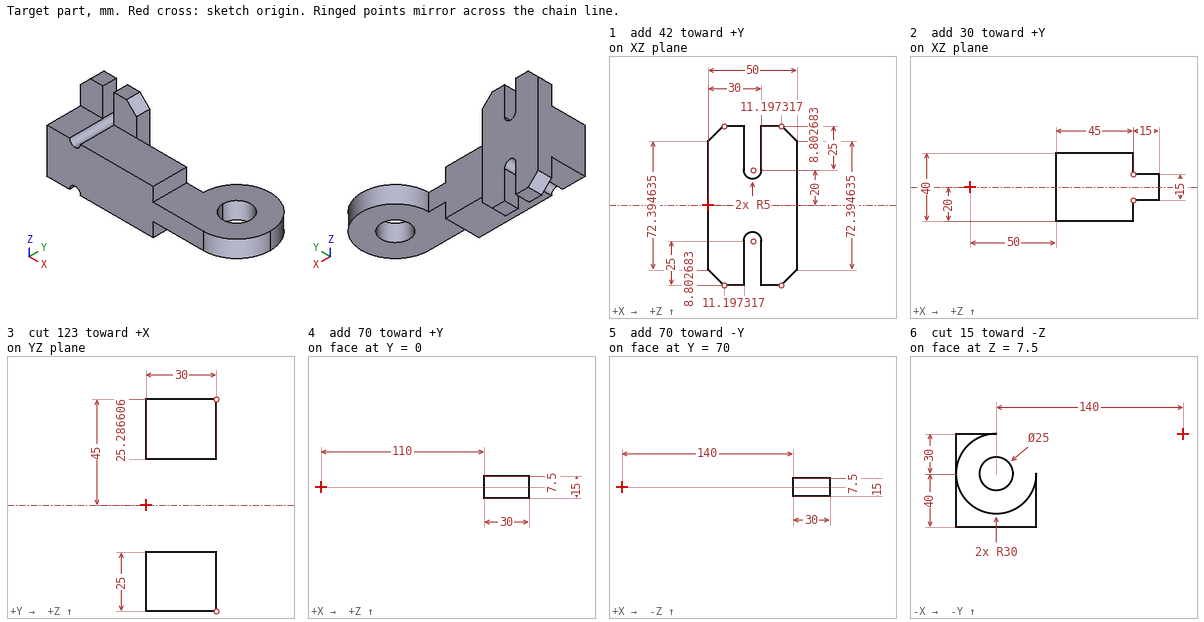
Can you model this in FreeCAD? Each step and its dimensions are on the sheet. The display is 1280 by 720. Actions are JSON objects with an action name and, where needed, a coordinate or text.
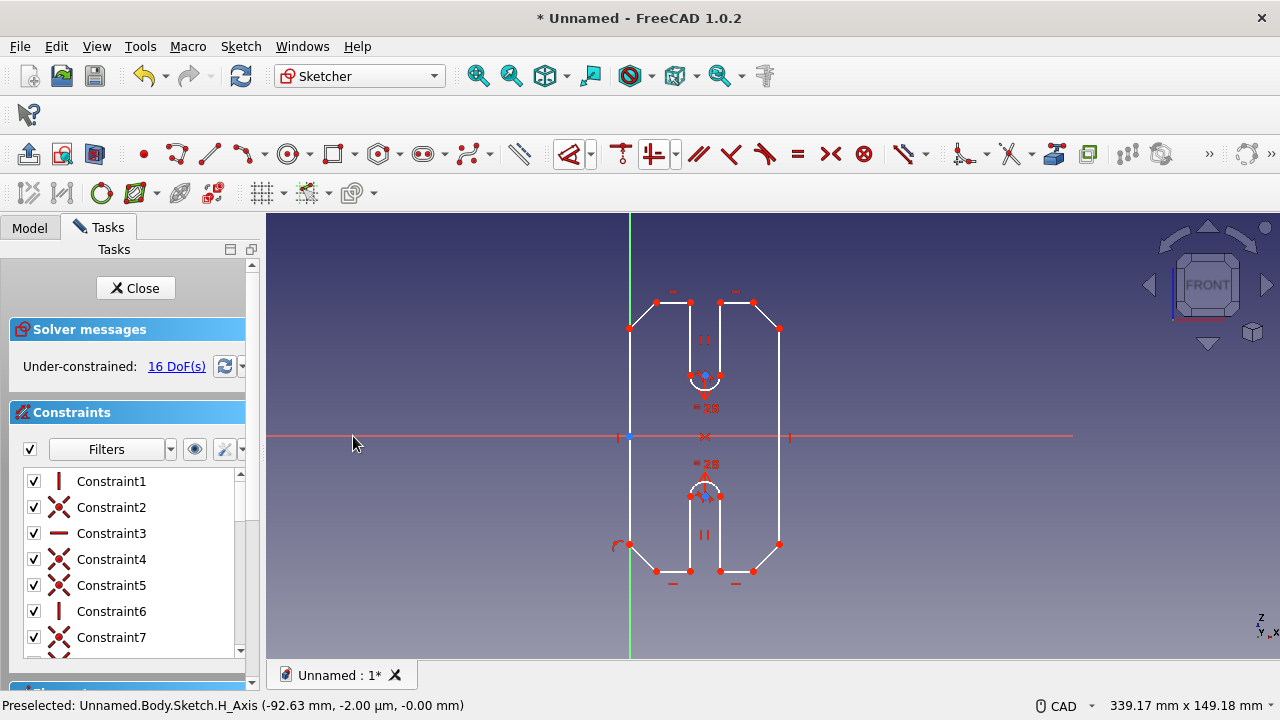
{"action": "left_click", "coordinate": [753, 303]}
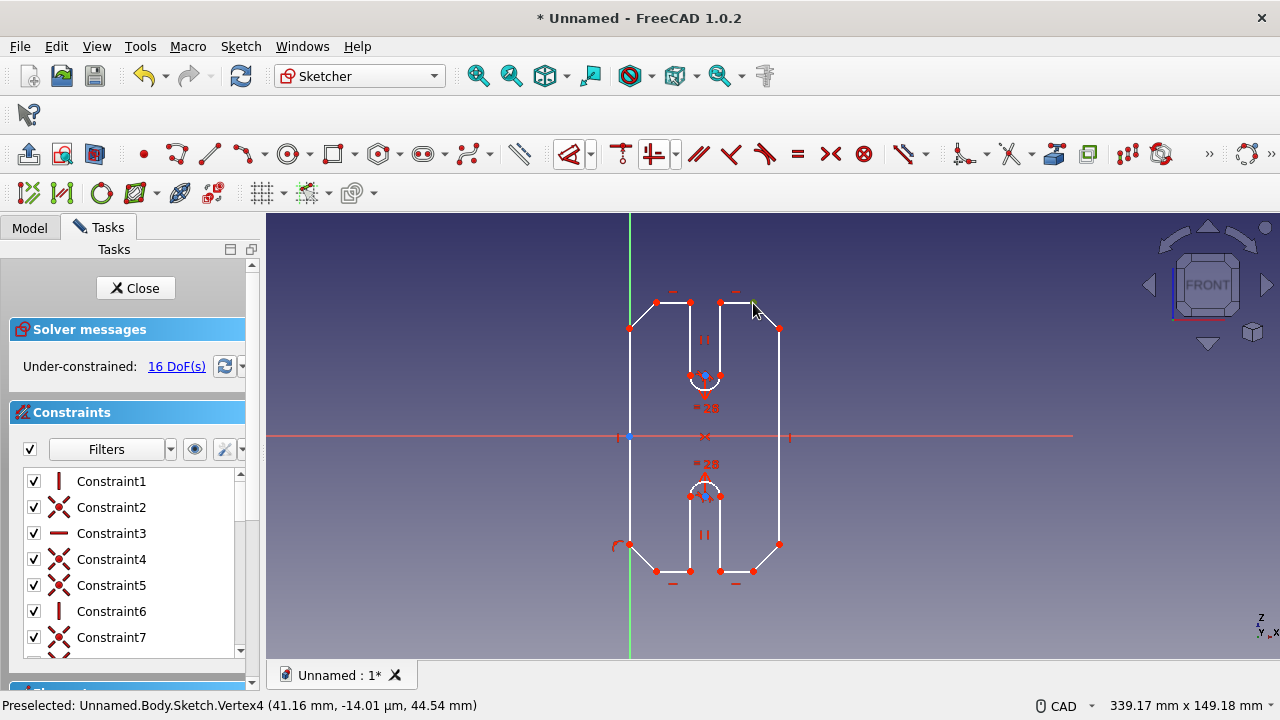
{"action": "left_click", "coordinate": [753, 572]}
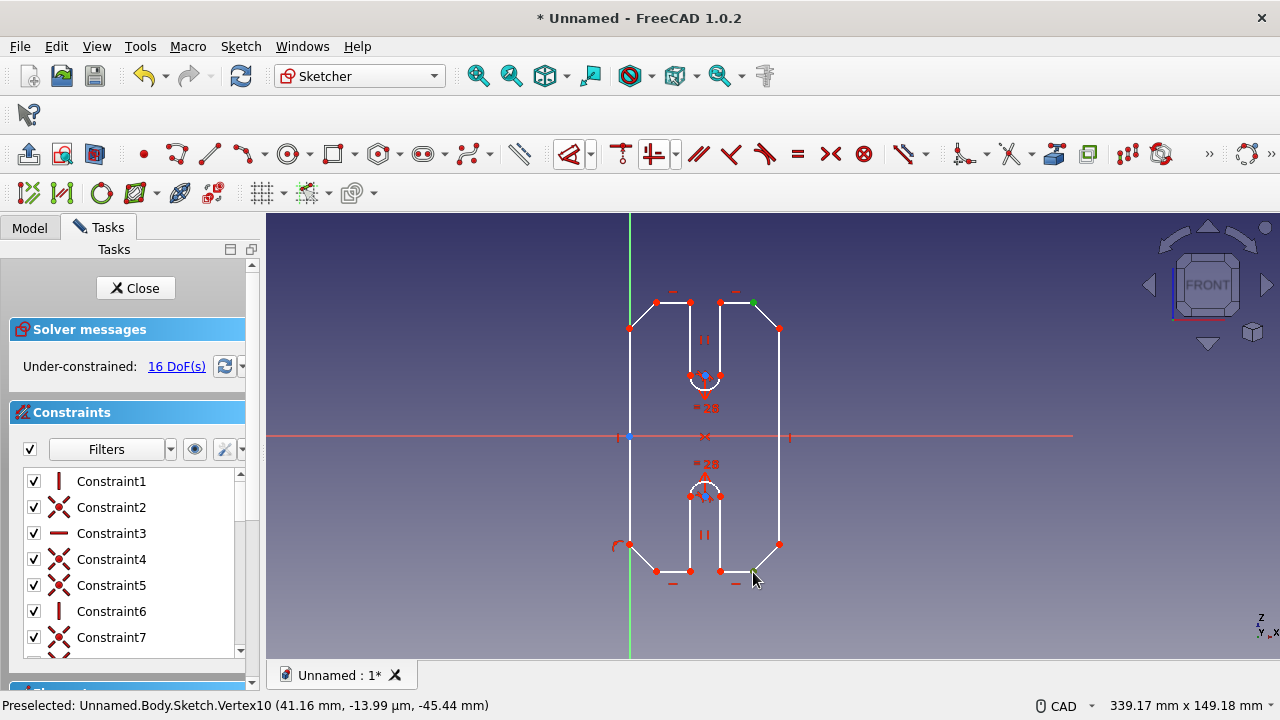
{"action": "left_click", "coordinate": [353, 436]}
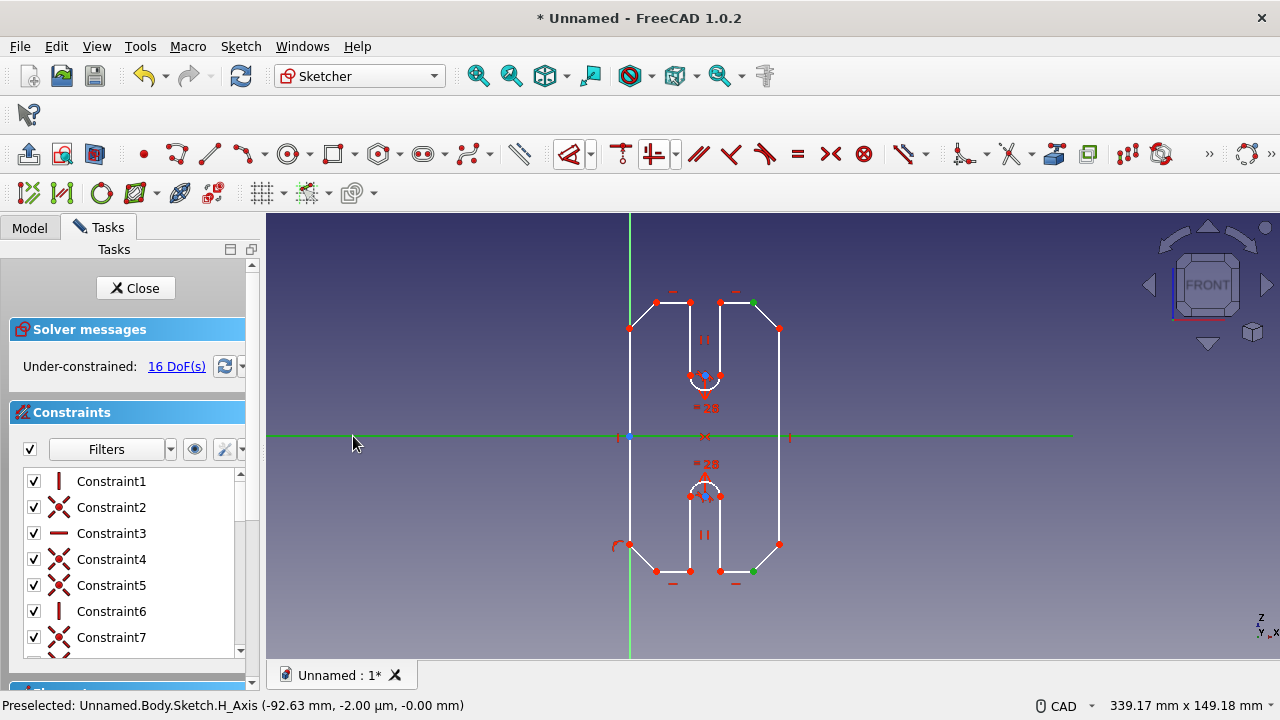
{"action": "left_click", "coordinate": [831, 154]}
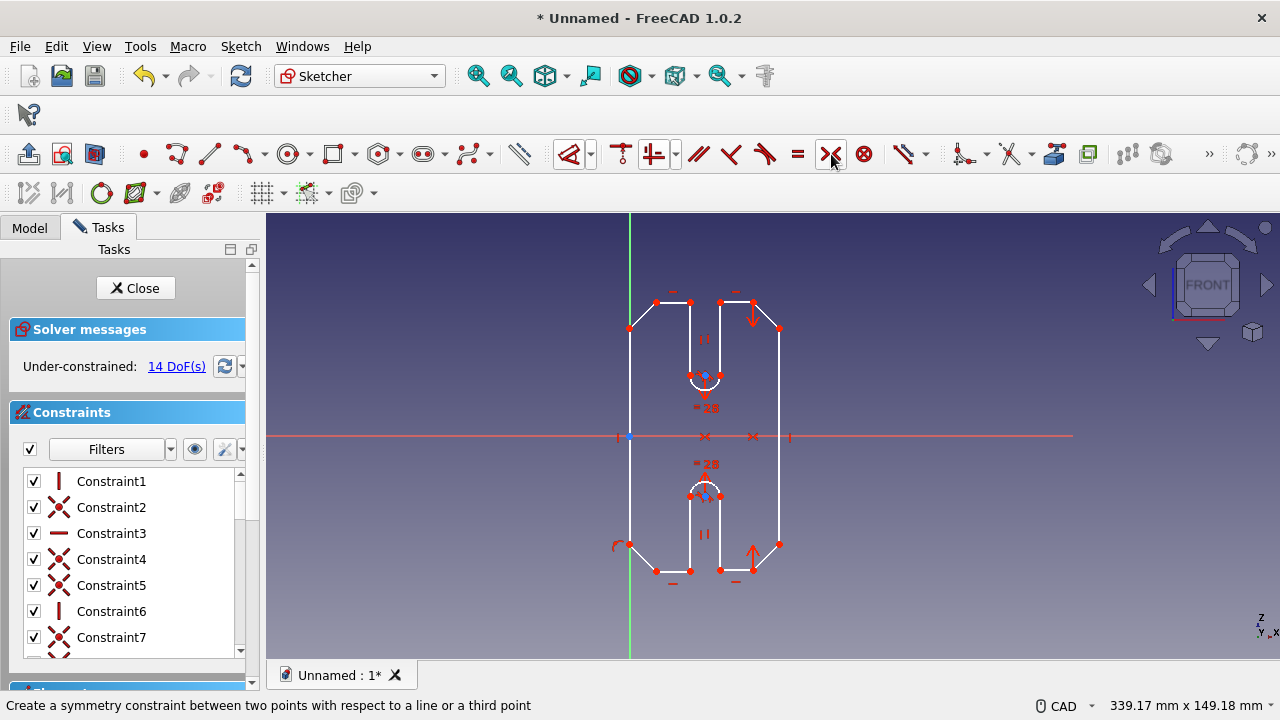
{"action": "left_click", "coordinate": [656, 572]}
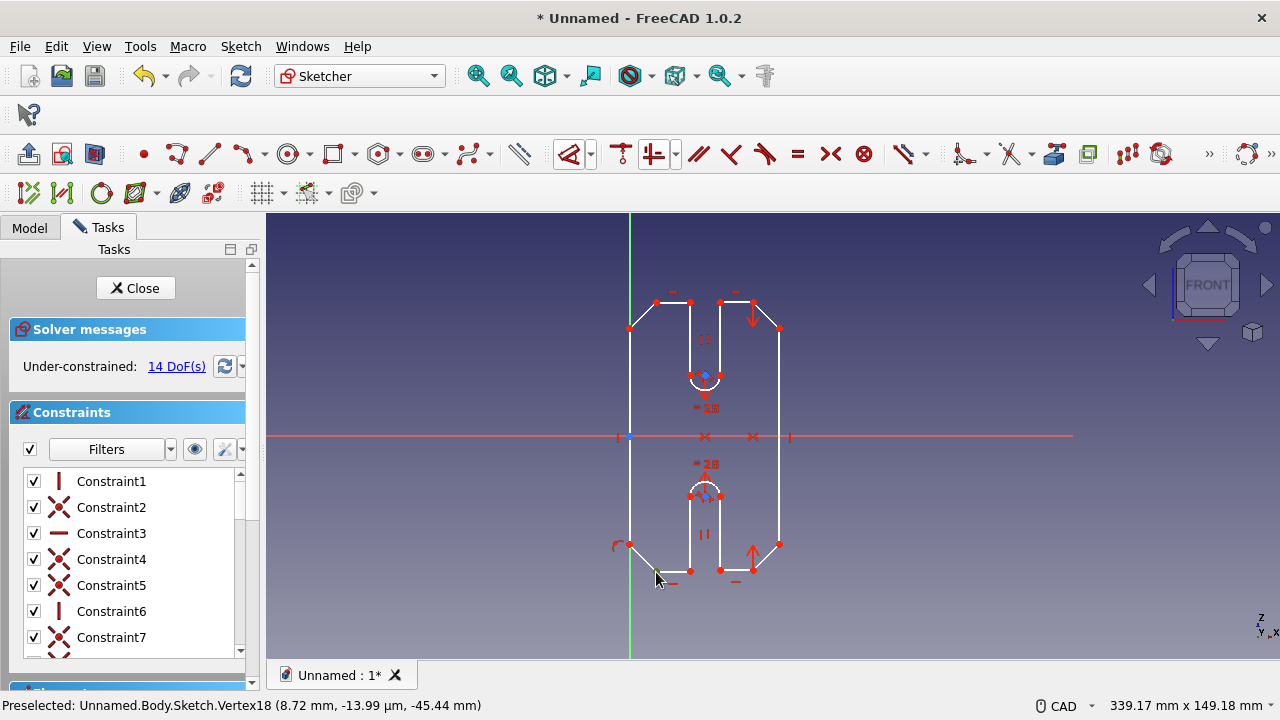
{"action": "left_click", "coordinate": [656, 303]}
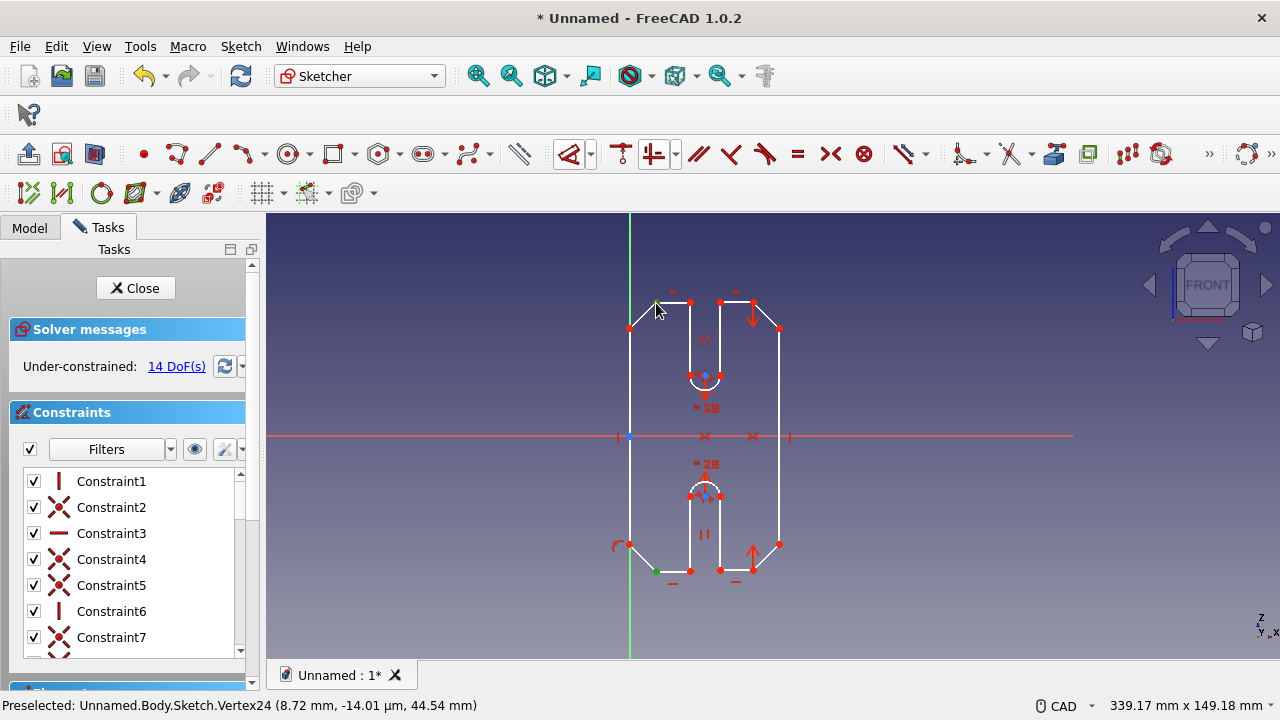
{"action": "left_click", "coordinate": [353, 436]}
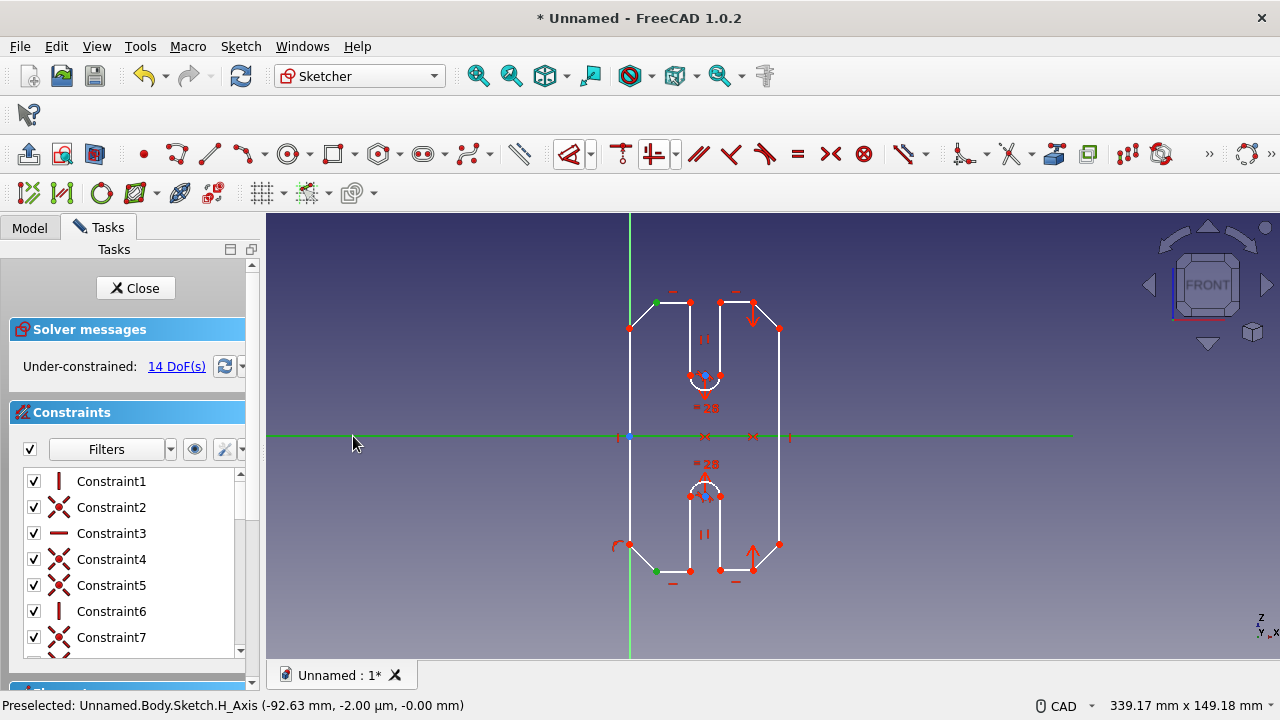
{"action": "left_click", "coordinate": [831, 154]}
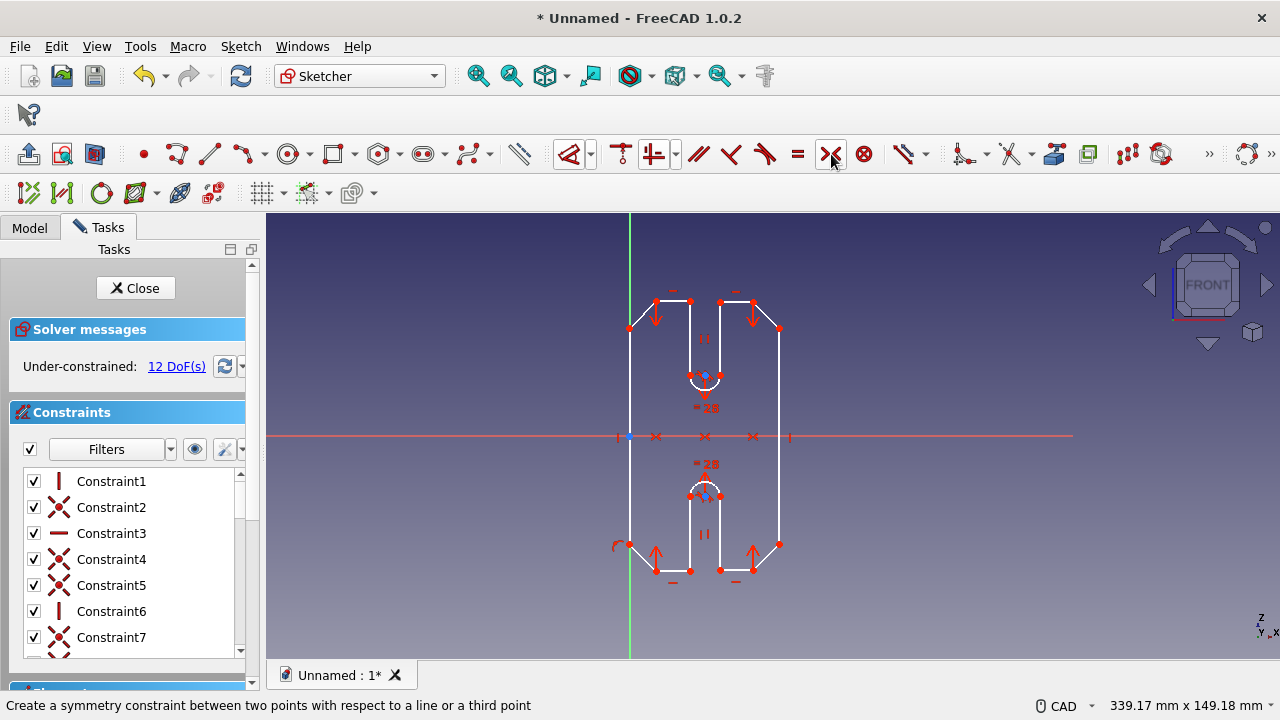
{"action": "left_click", "coordinate": [568, 154]}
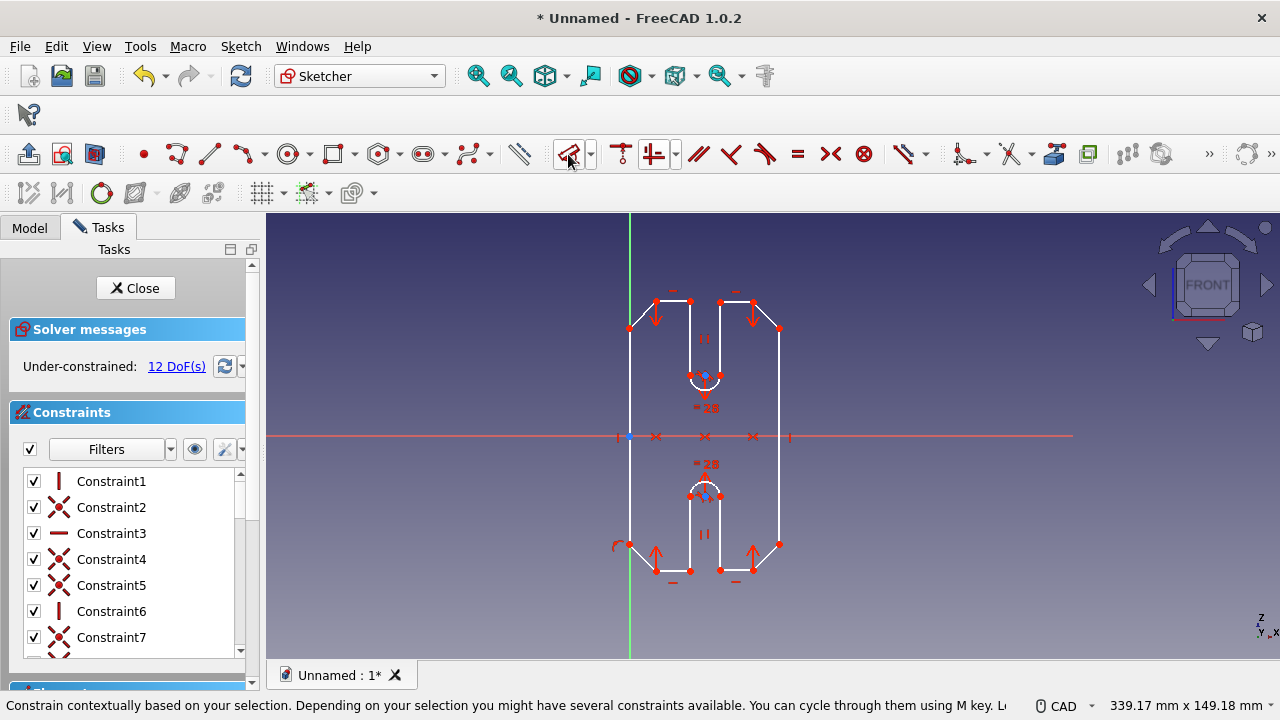
{"action": "scroll", "coordinate": [714, 485], "scroll_direction": "up", "scroll_amount": 5}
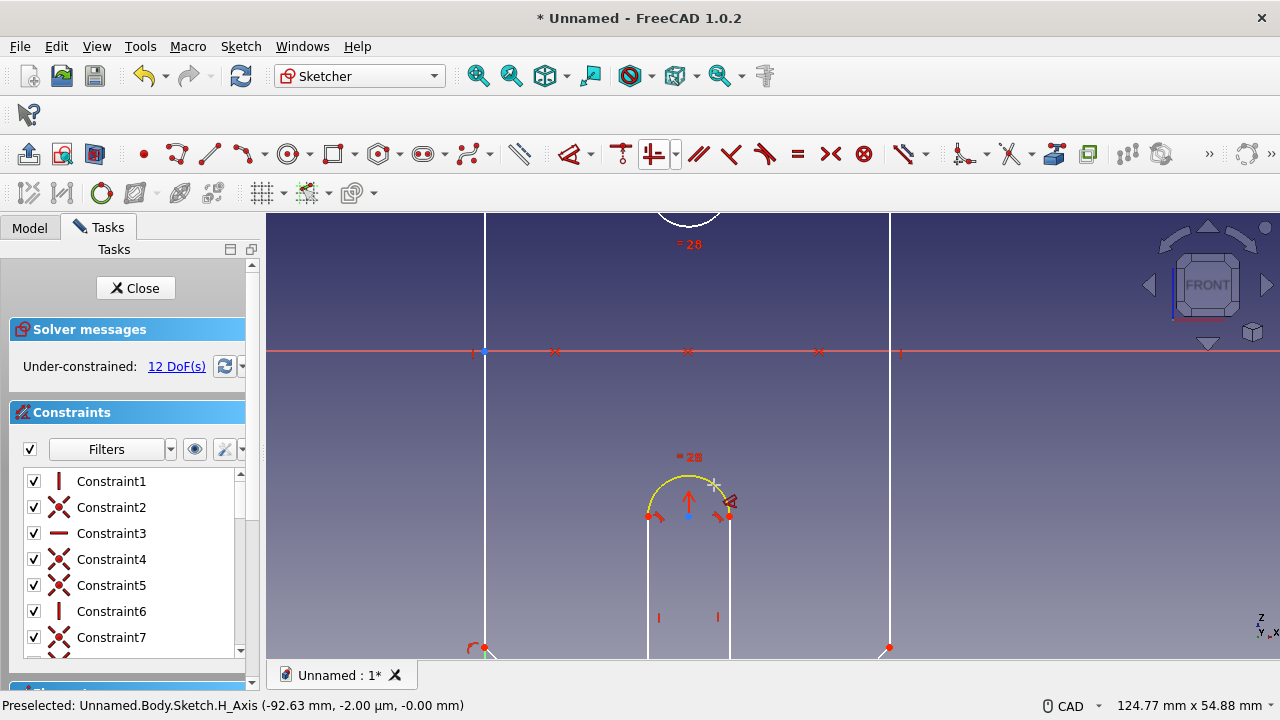
{"action": "left_click", "coordinate": [713, 484]}
{"action": "left_click", "coordinate": [732, 458]}